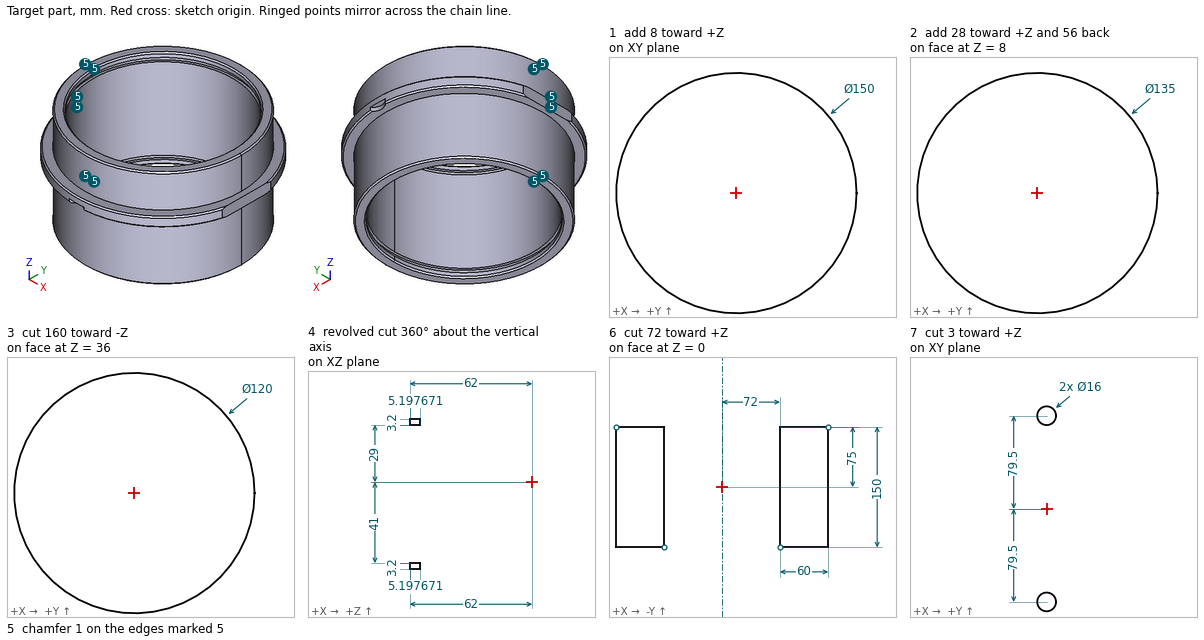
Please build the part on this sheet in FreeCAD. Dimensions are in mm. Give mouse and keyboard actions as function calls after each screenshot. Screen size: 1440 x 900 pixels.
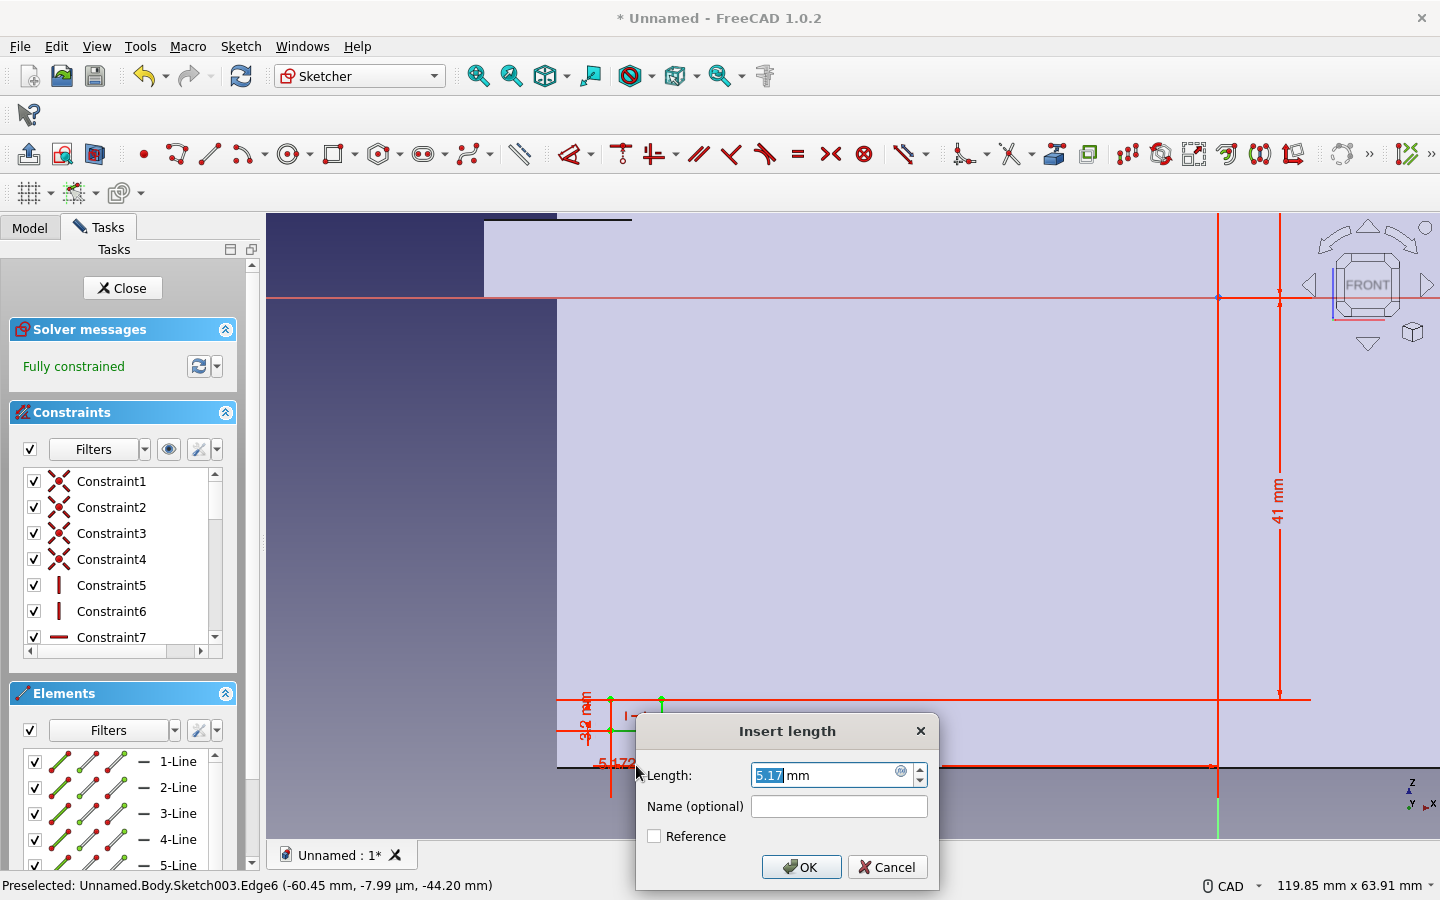
text(5.197671)
key(Return)
key(Escape)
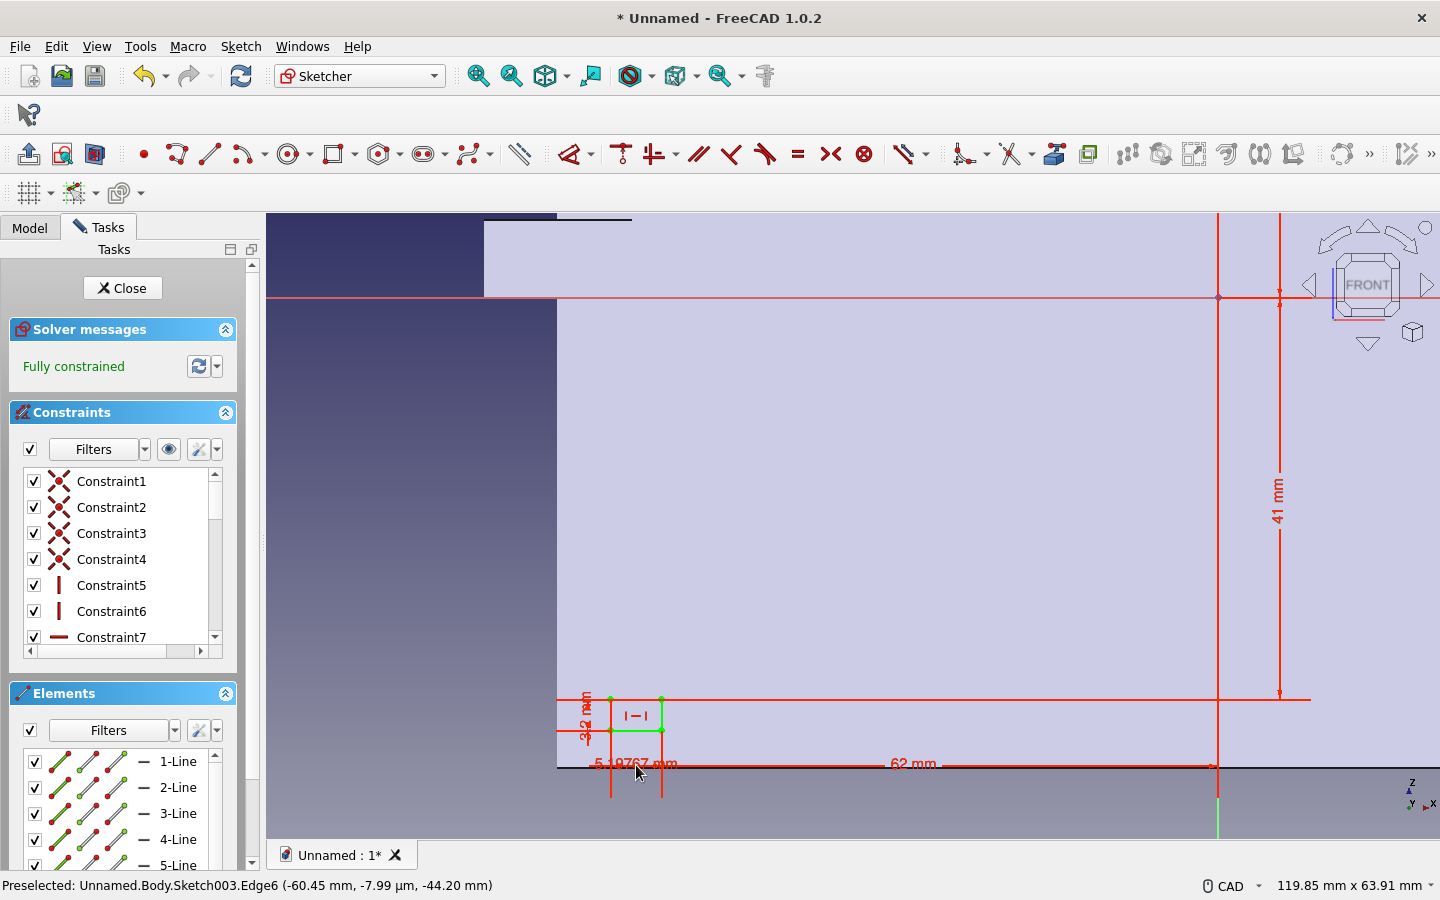
click(123, 288)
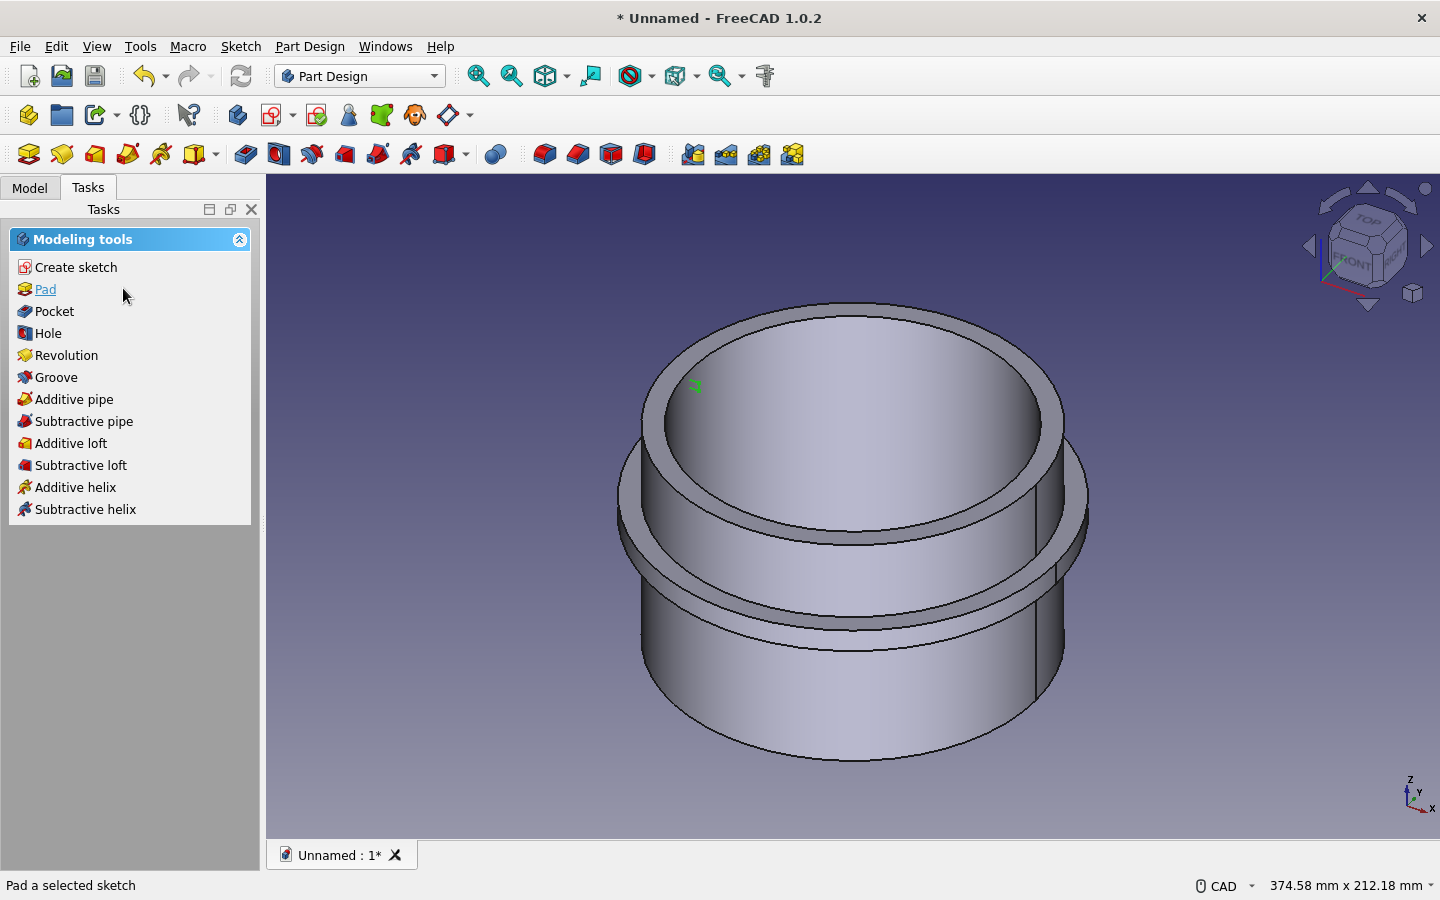
click(312, 154)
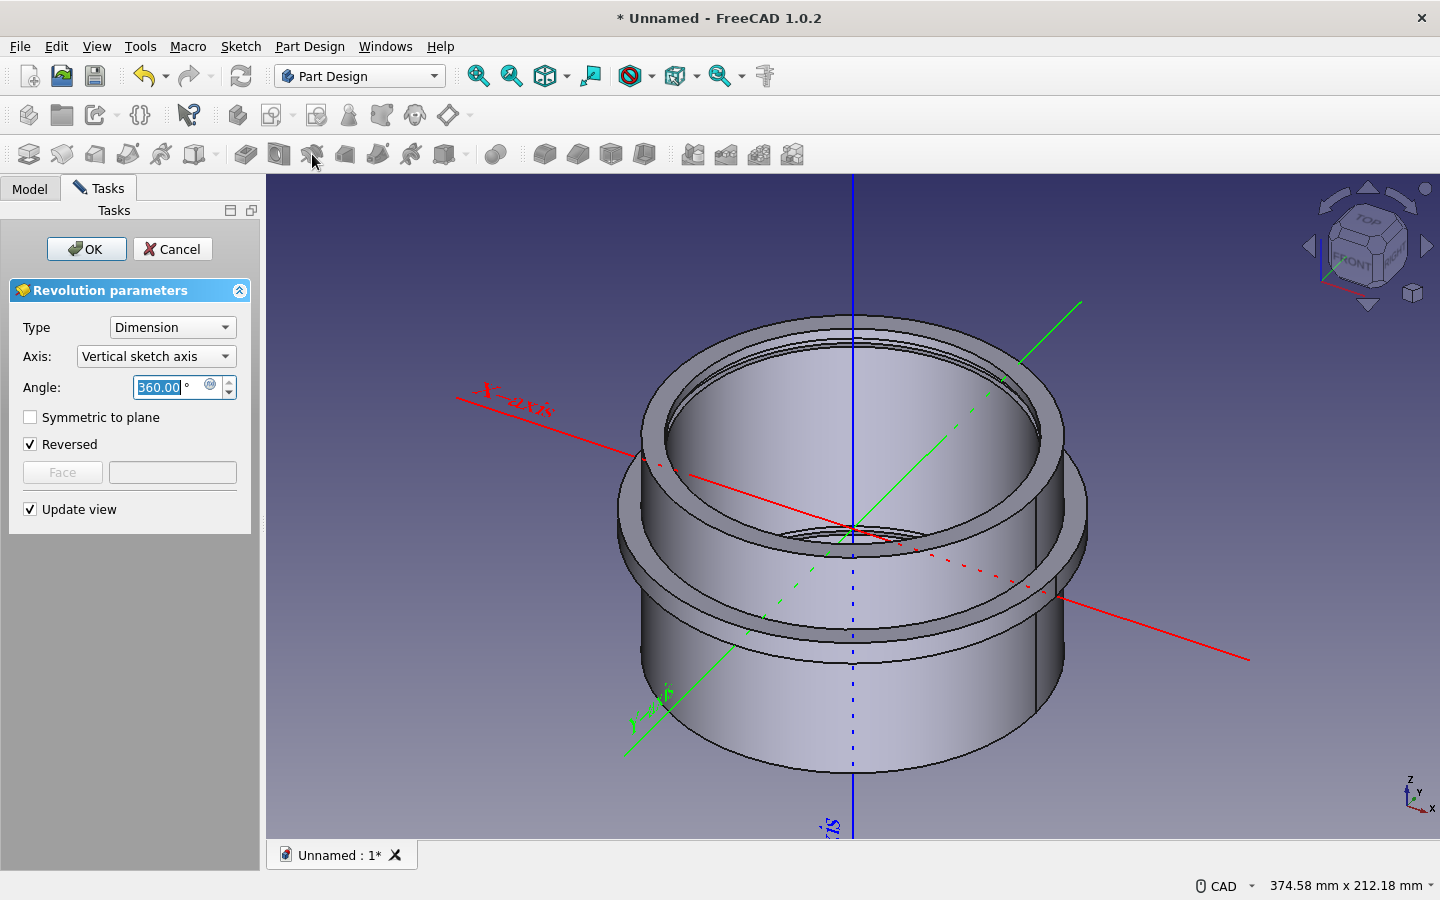
click(87, 249)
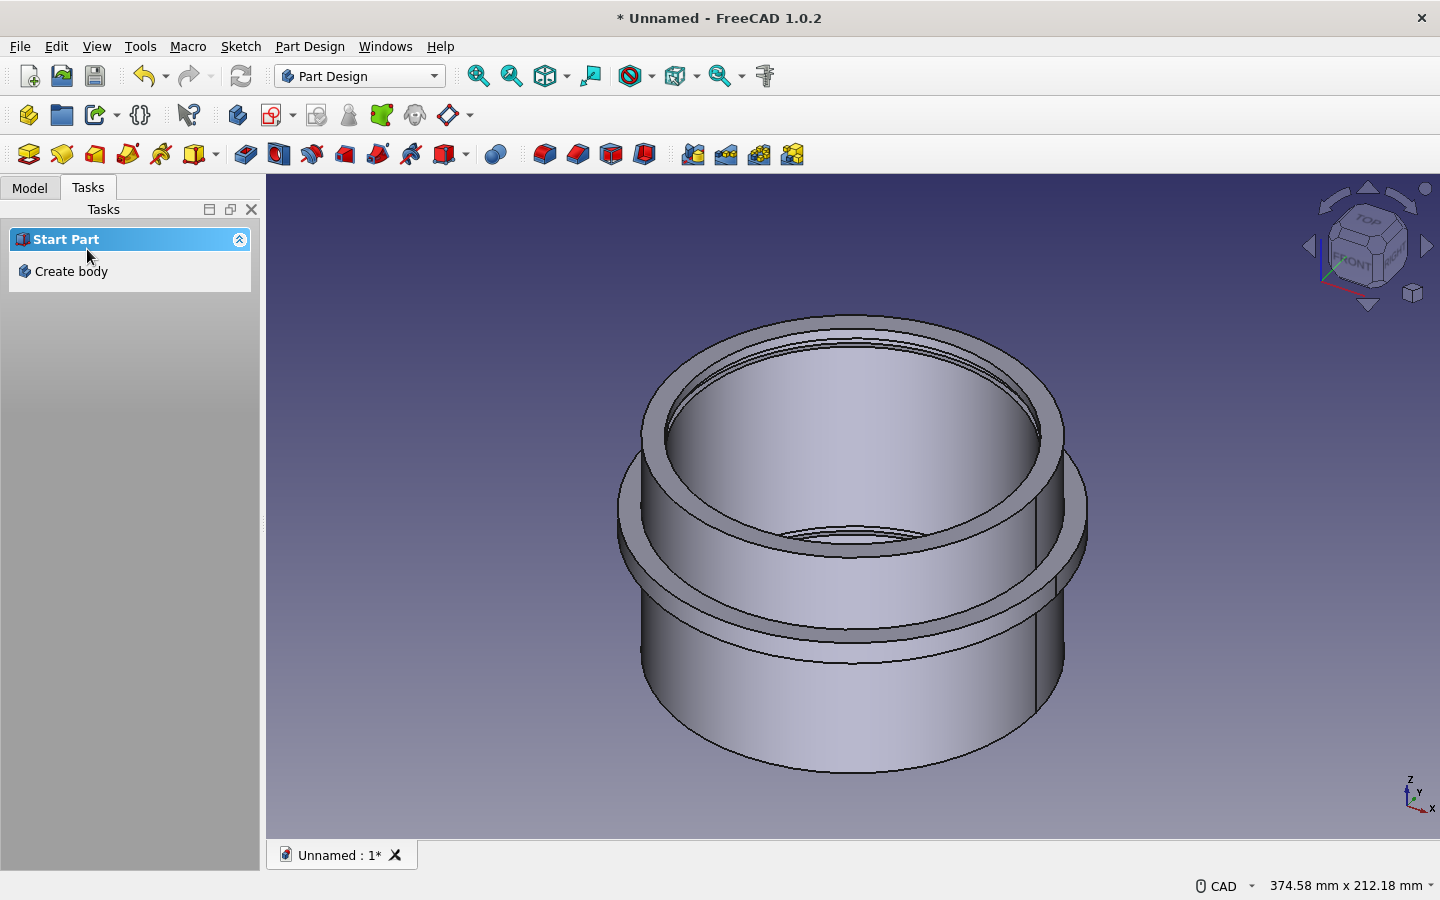
click(690, 381)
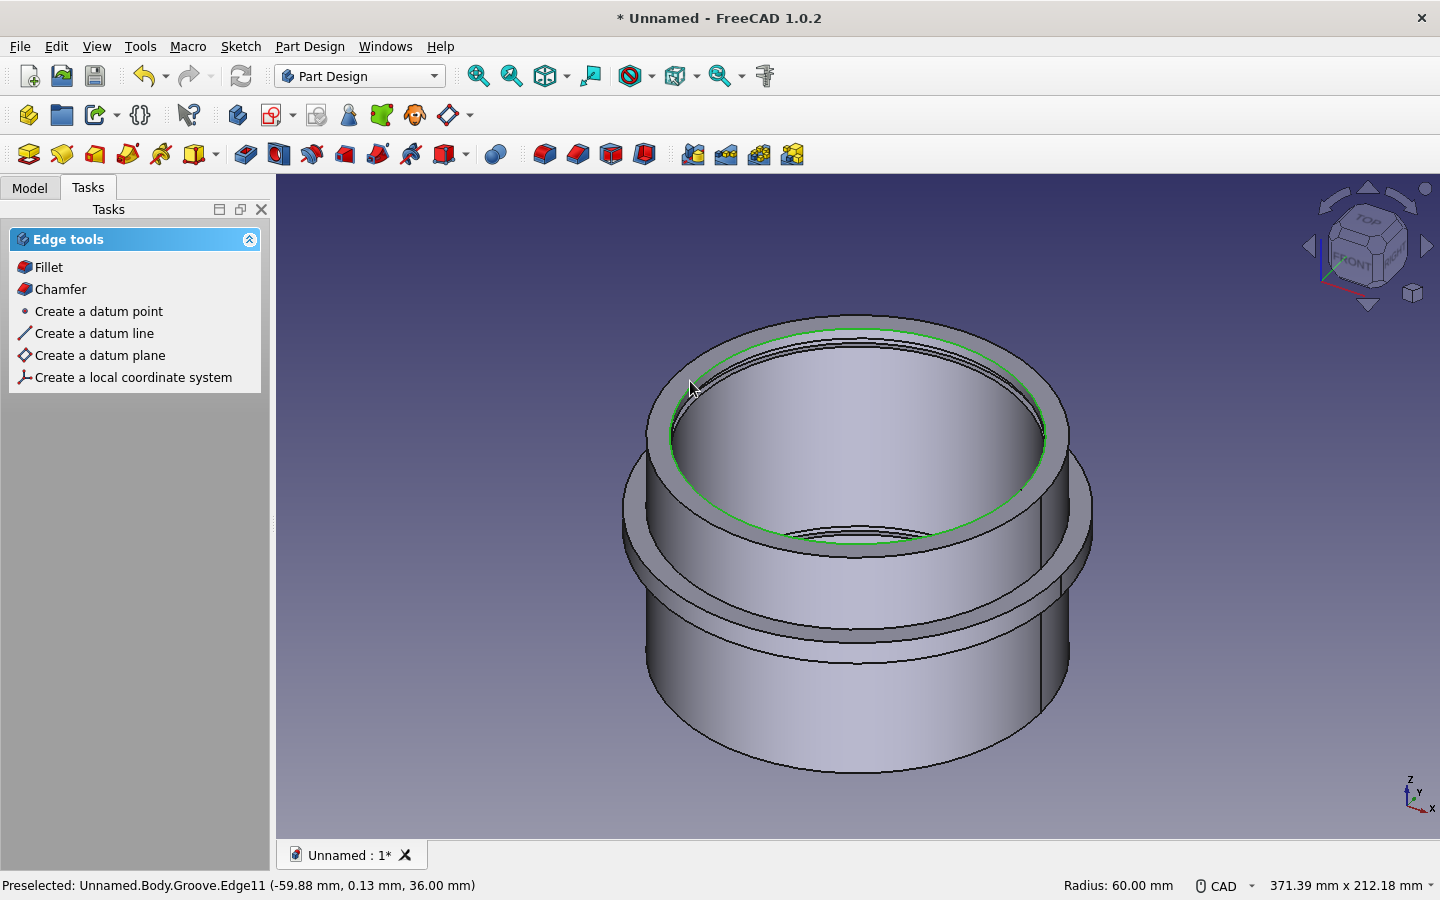
click(624, 521, ctrl)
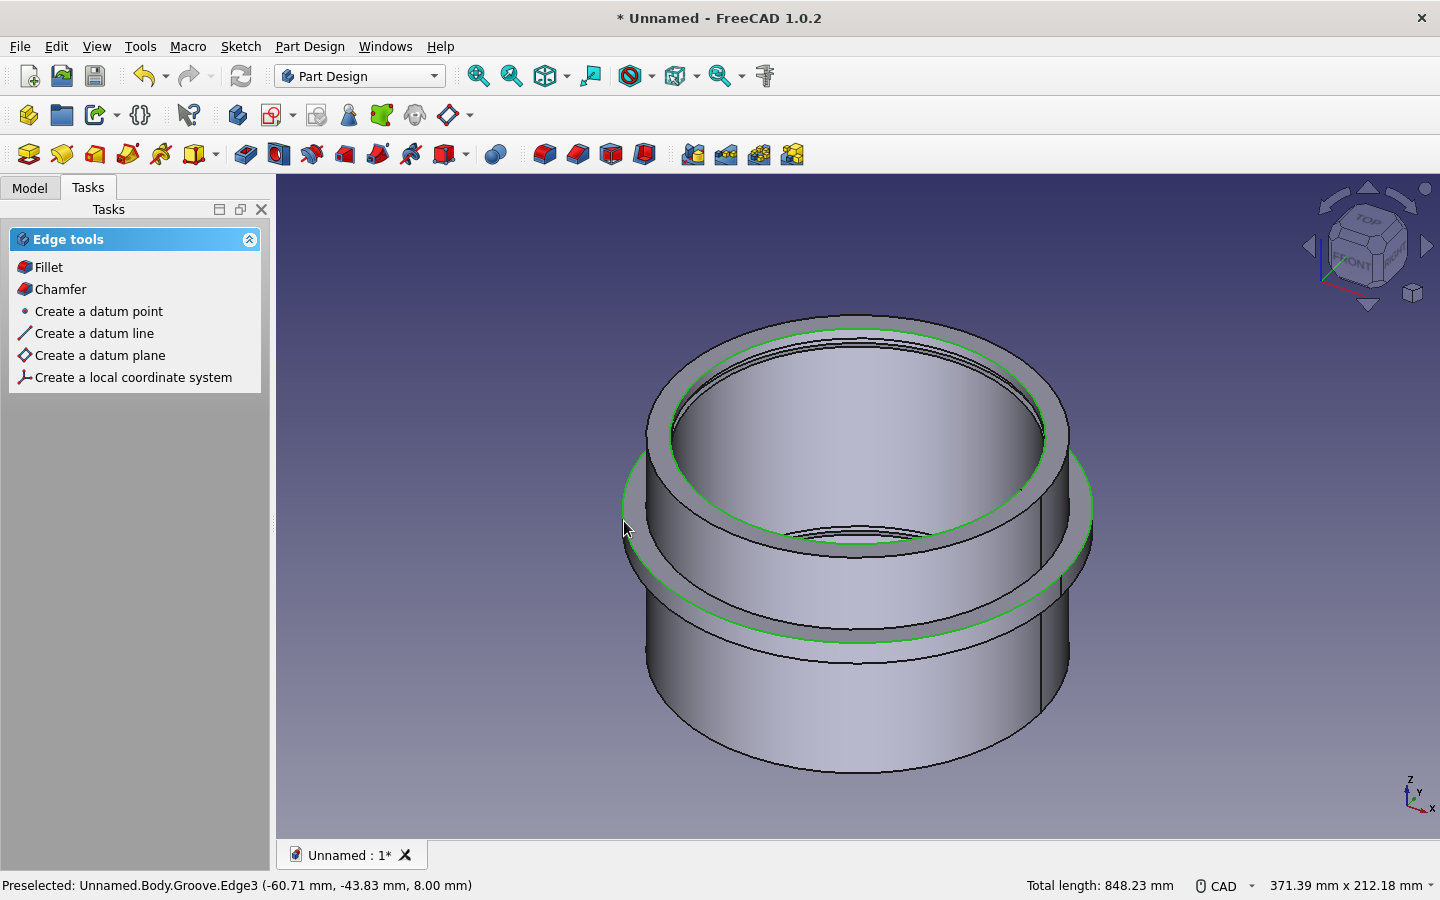
click(647, 448, ctrl)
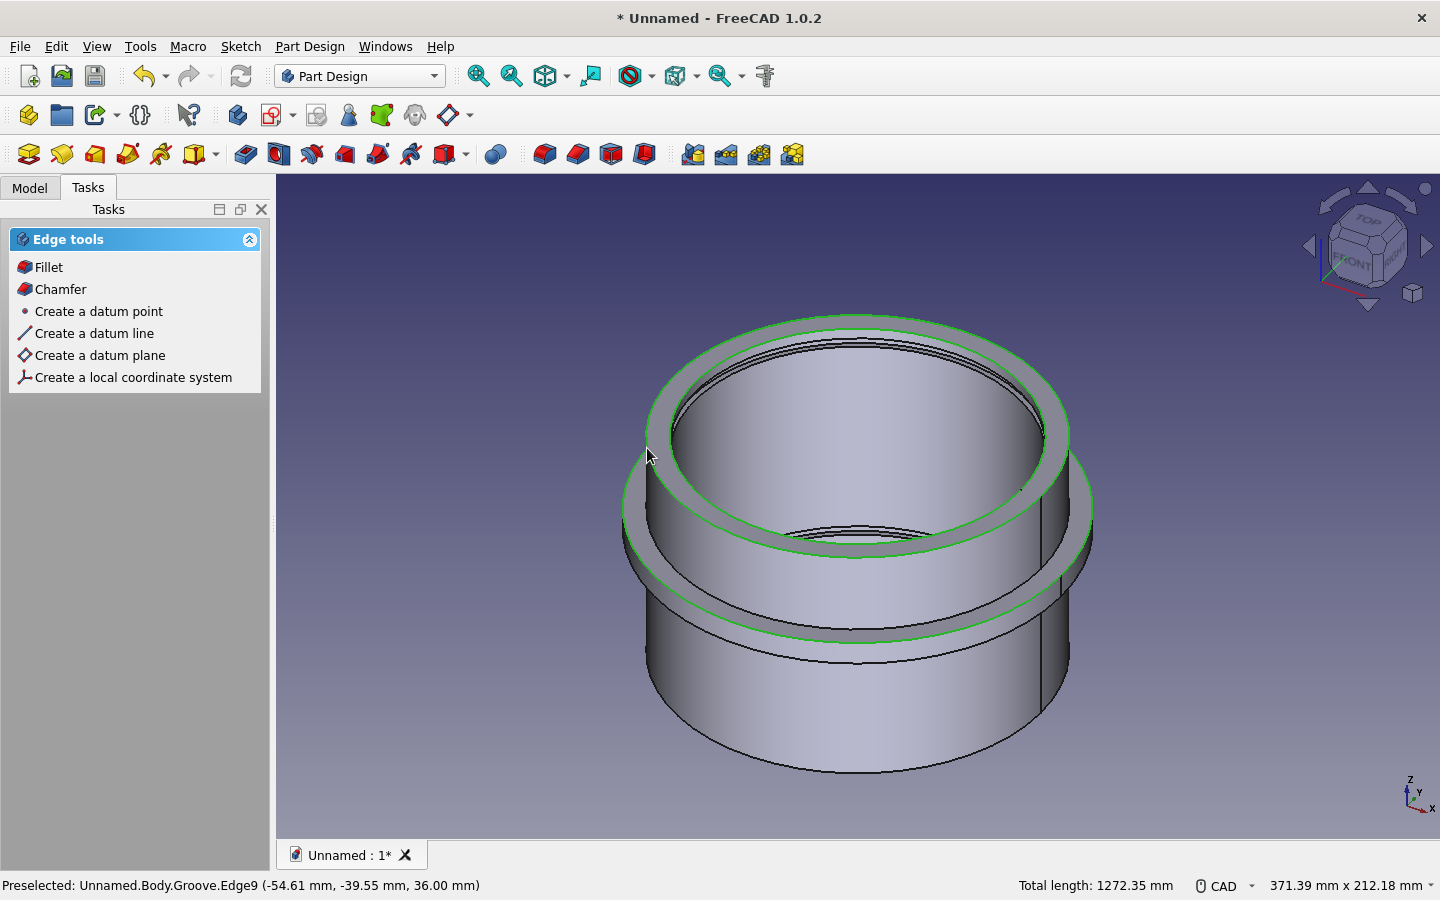
key(0)